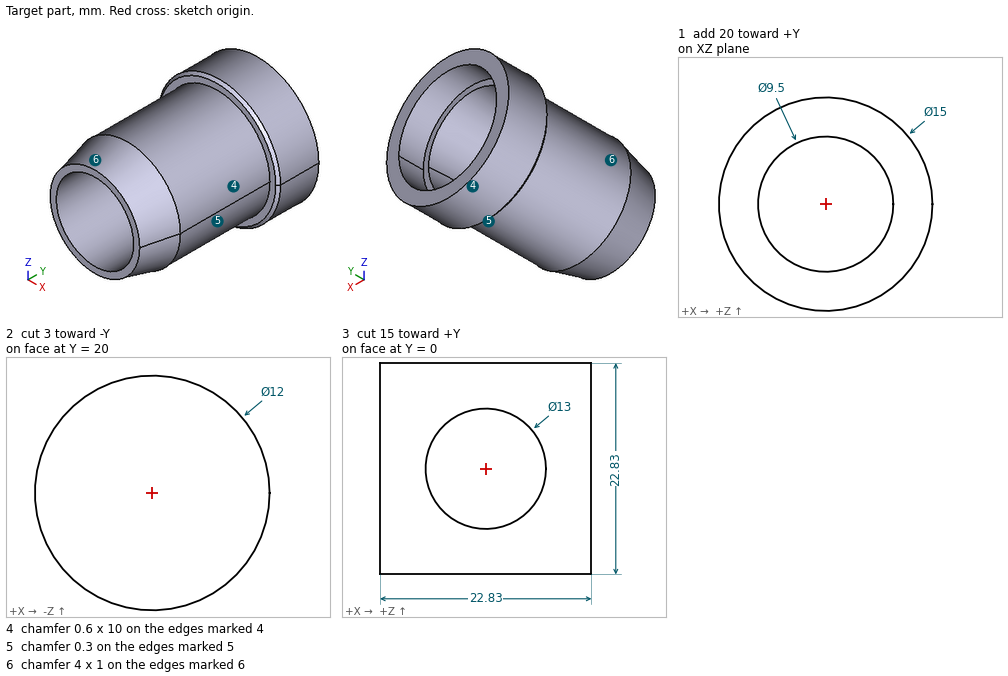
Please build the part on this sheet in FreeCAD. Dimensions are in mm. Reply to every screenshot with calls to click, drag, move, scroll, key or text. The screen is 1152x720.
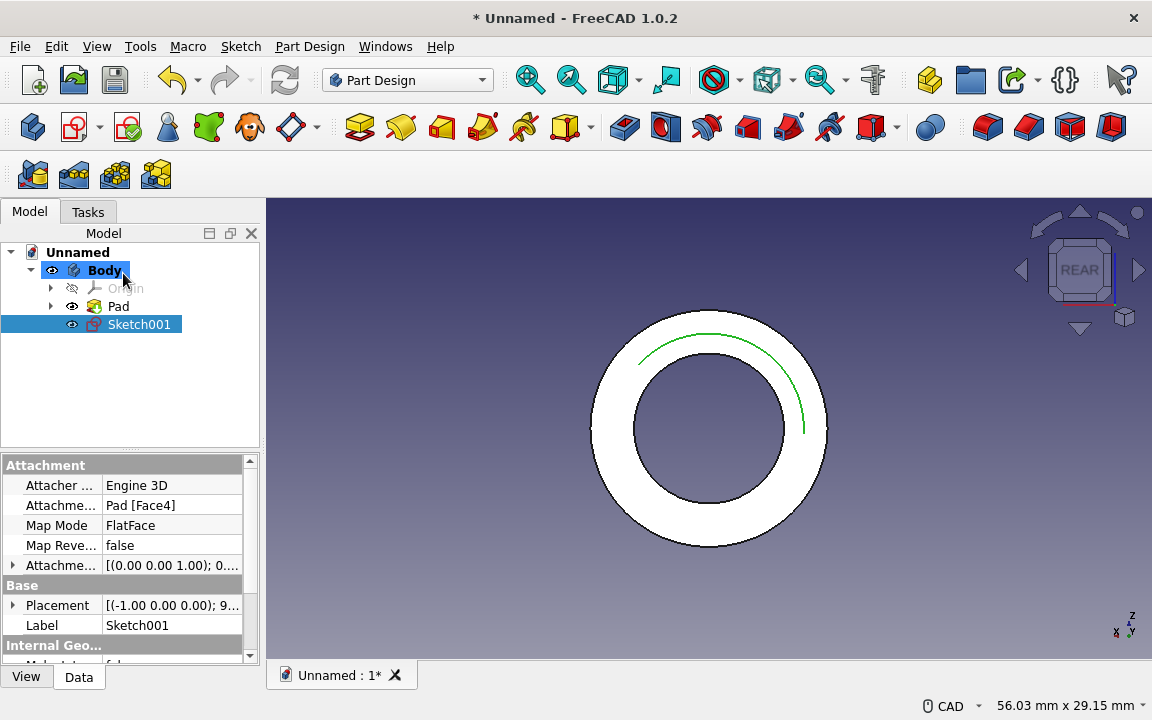
click(625, 128)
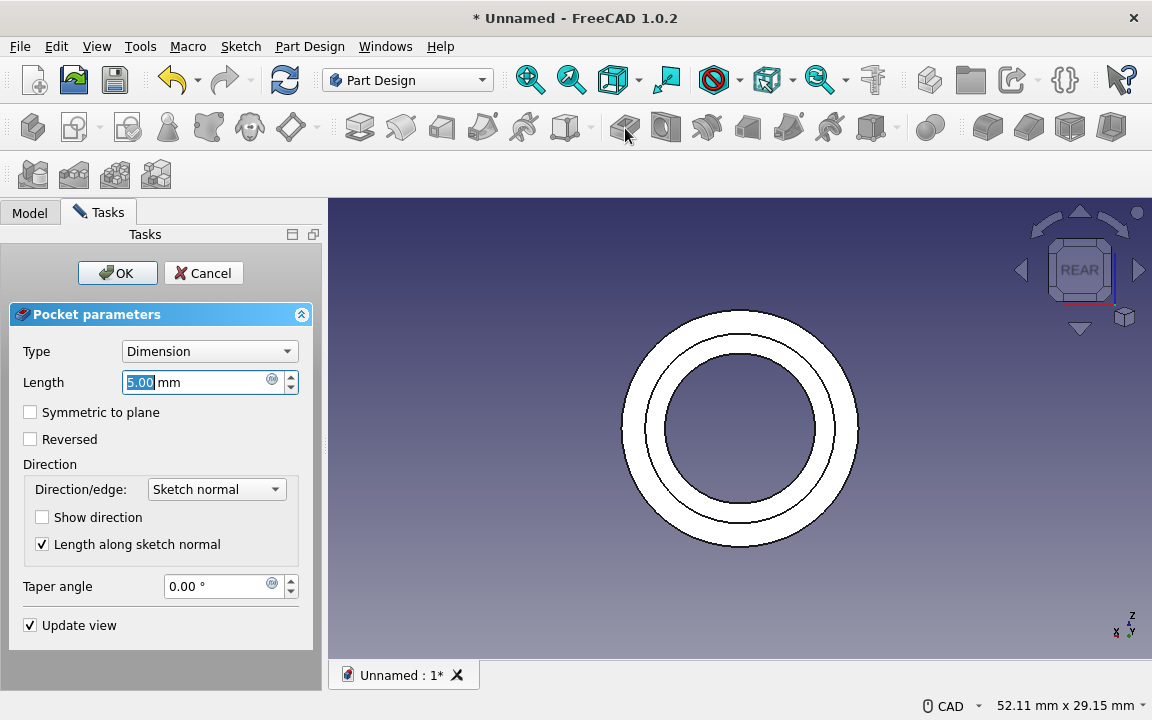
text(3)
key(Tab)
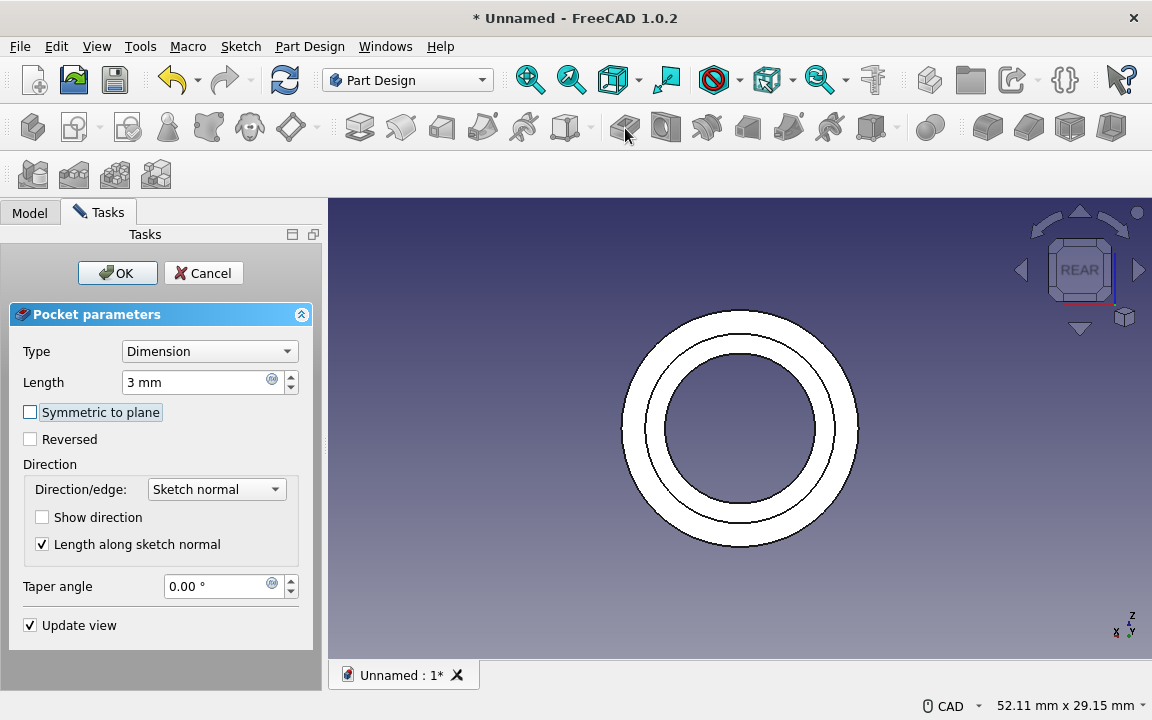
click(118, 273)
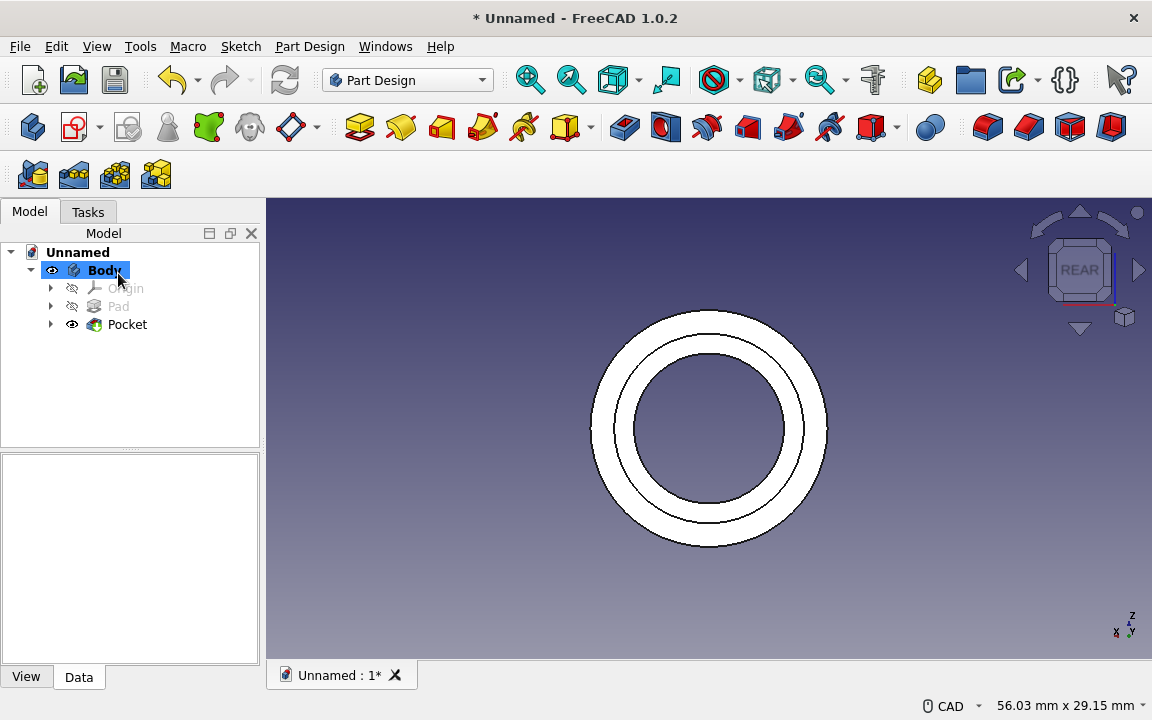
key(0)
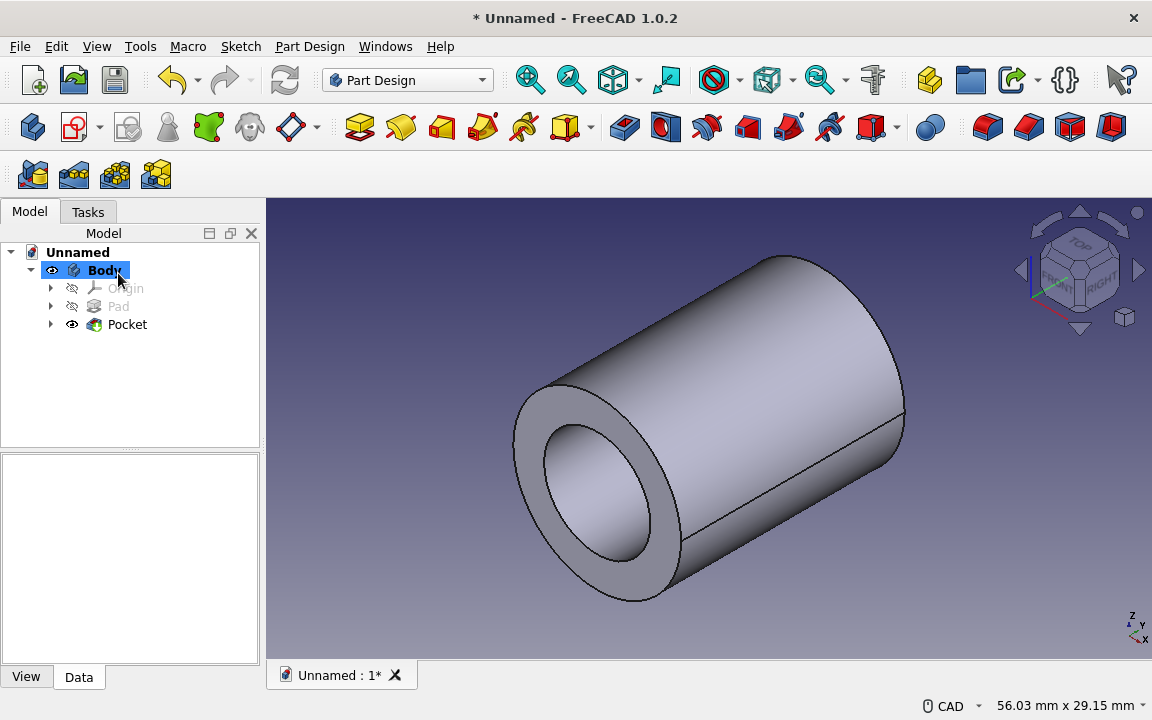
click(645, 464)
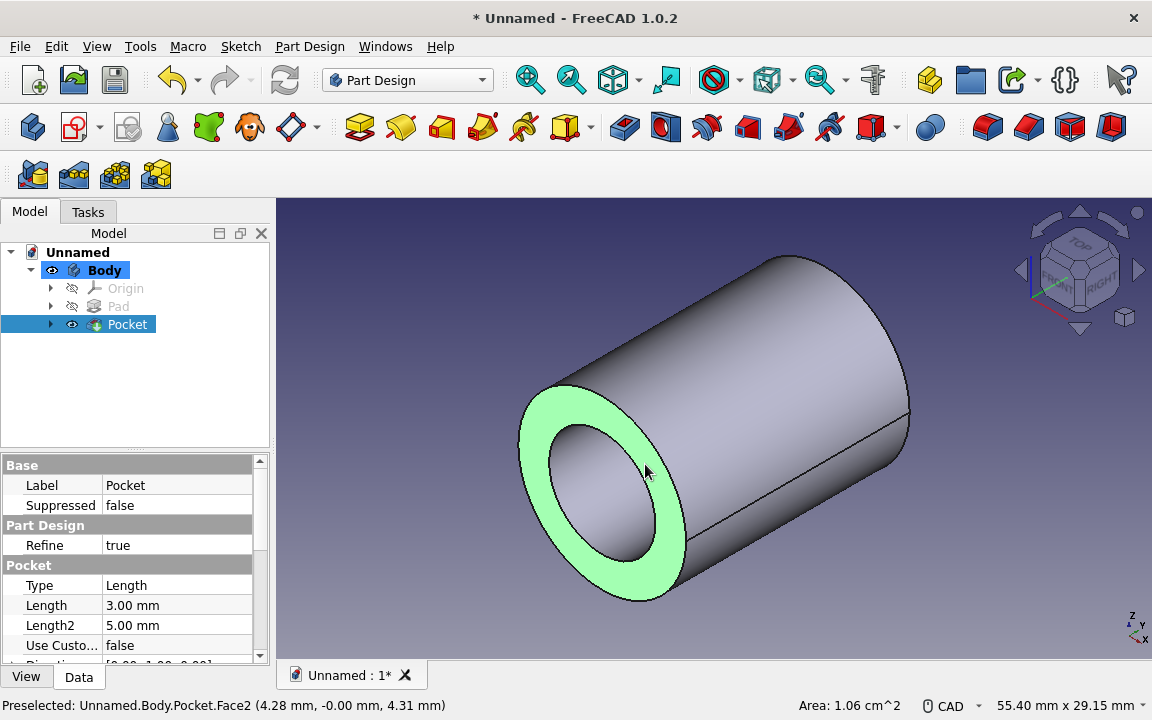
click(74, 128)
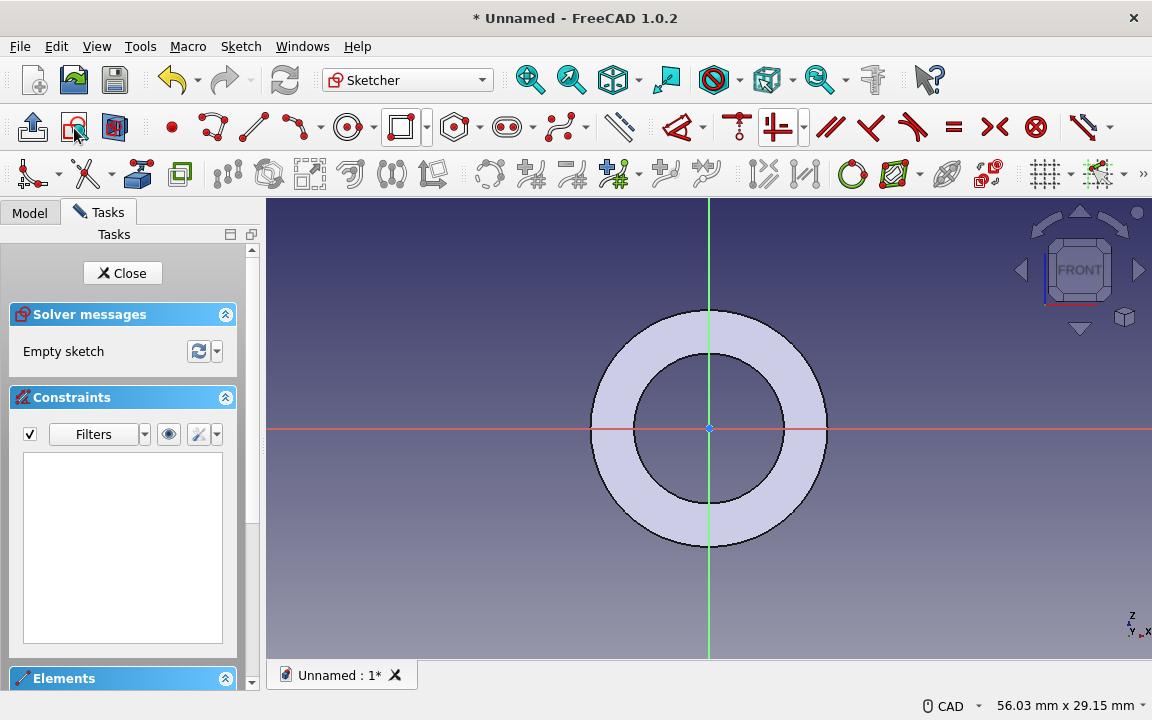
scroll(331, 428, down, 1)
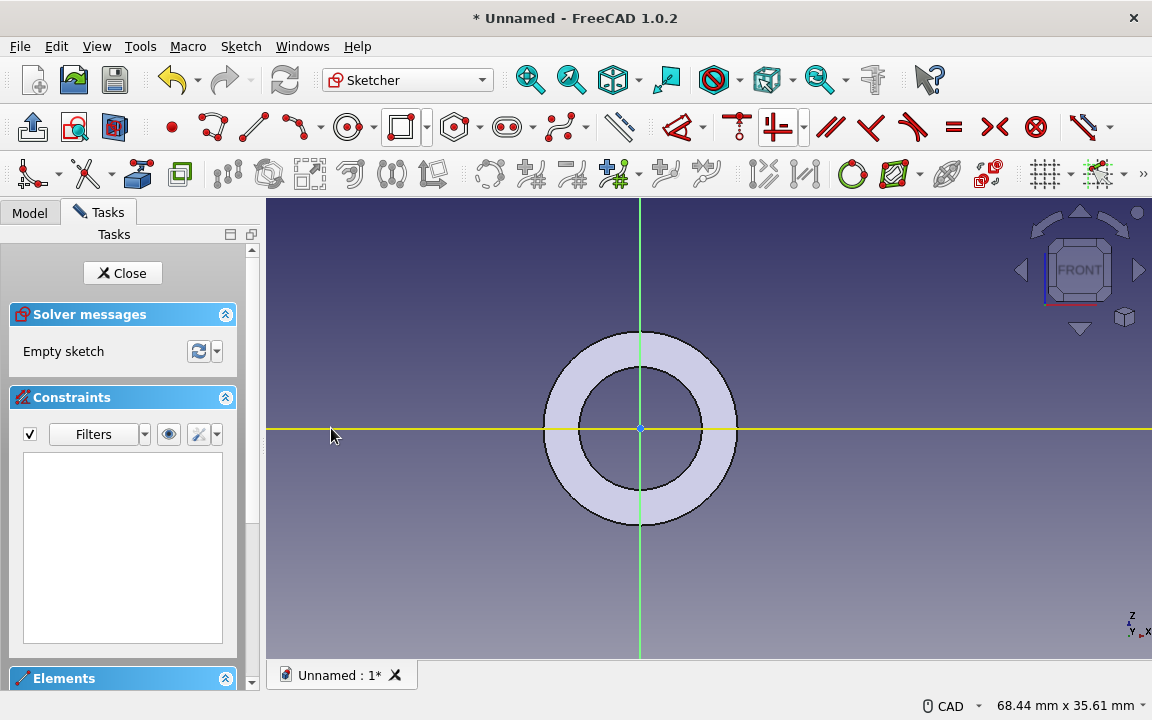
click(426, 128)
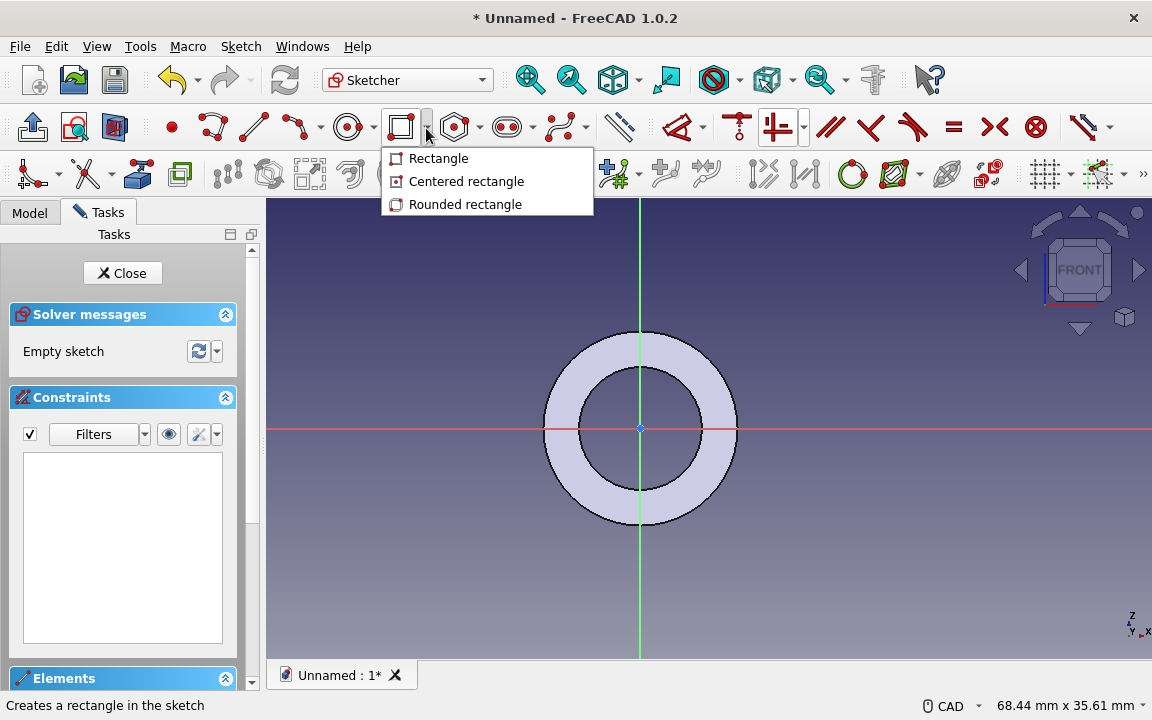
click(488, 182)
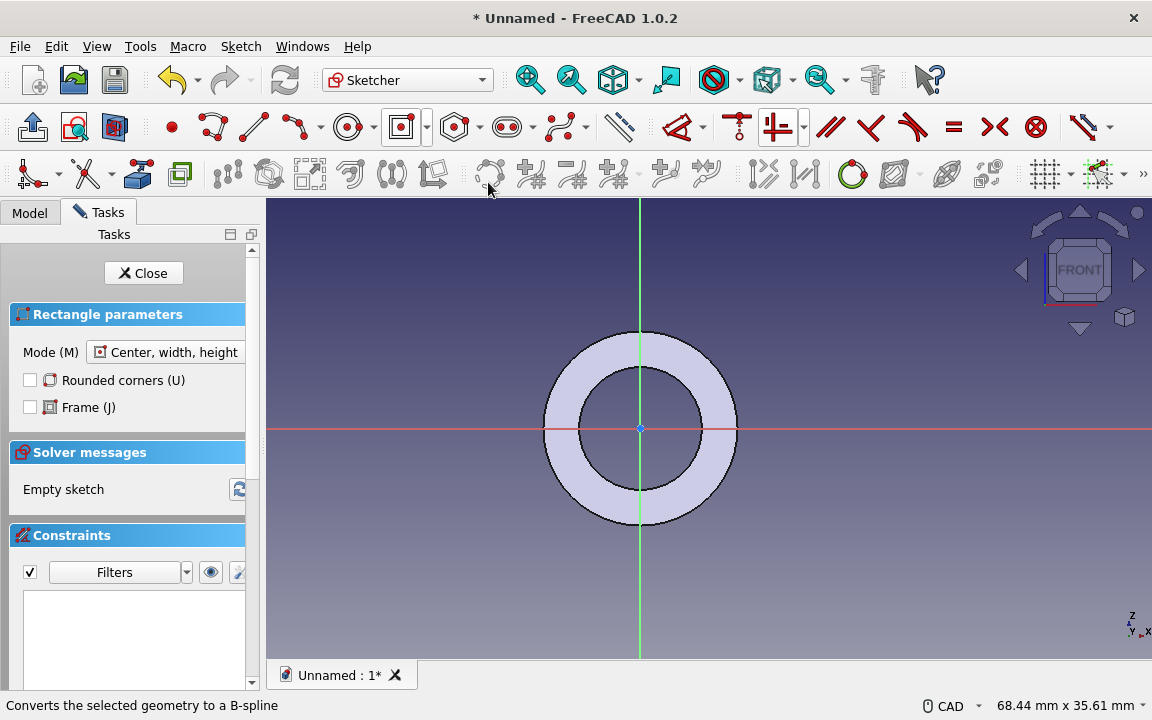
click(640, 429)
move(788, 281)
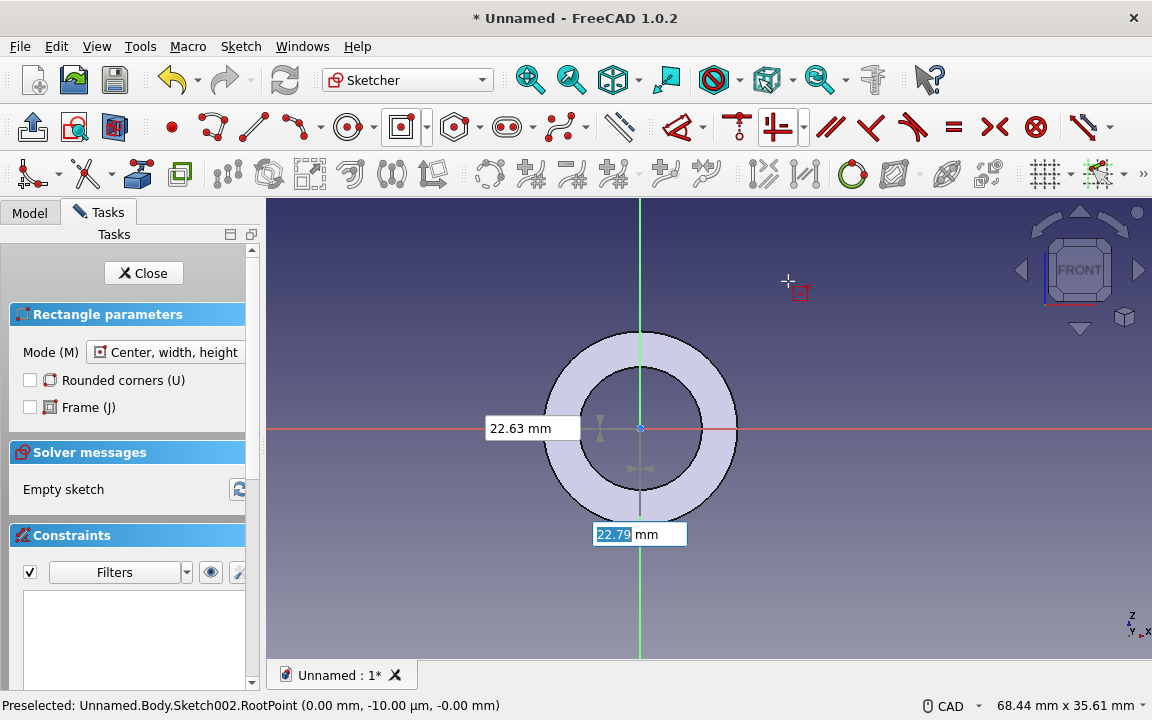
text(22.83)
key(Tab)
text(22.83)
key(Return)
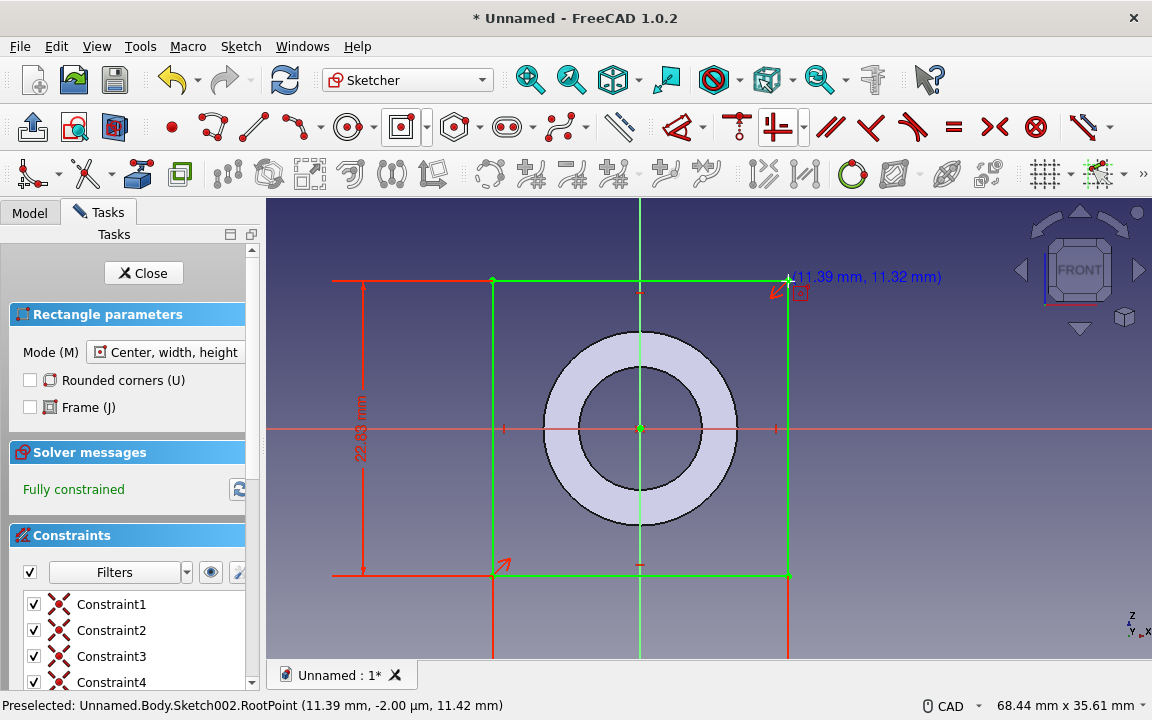
click(348, 128)